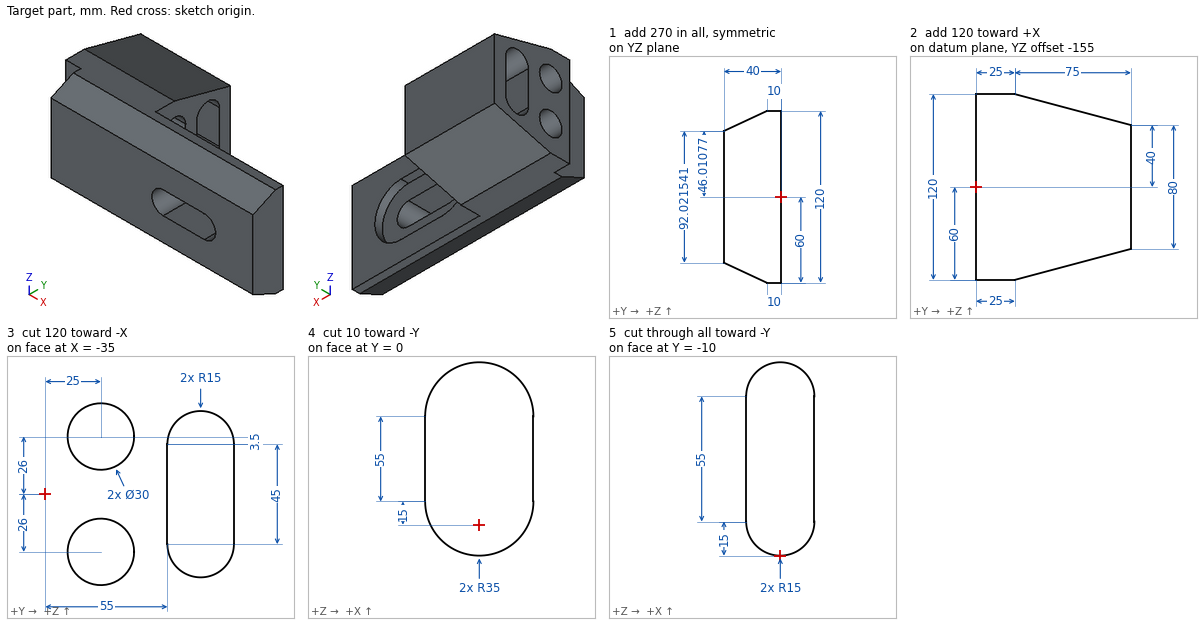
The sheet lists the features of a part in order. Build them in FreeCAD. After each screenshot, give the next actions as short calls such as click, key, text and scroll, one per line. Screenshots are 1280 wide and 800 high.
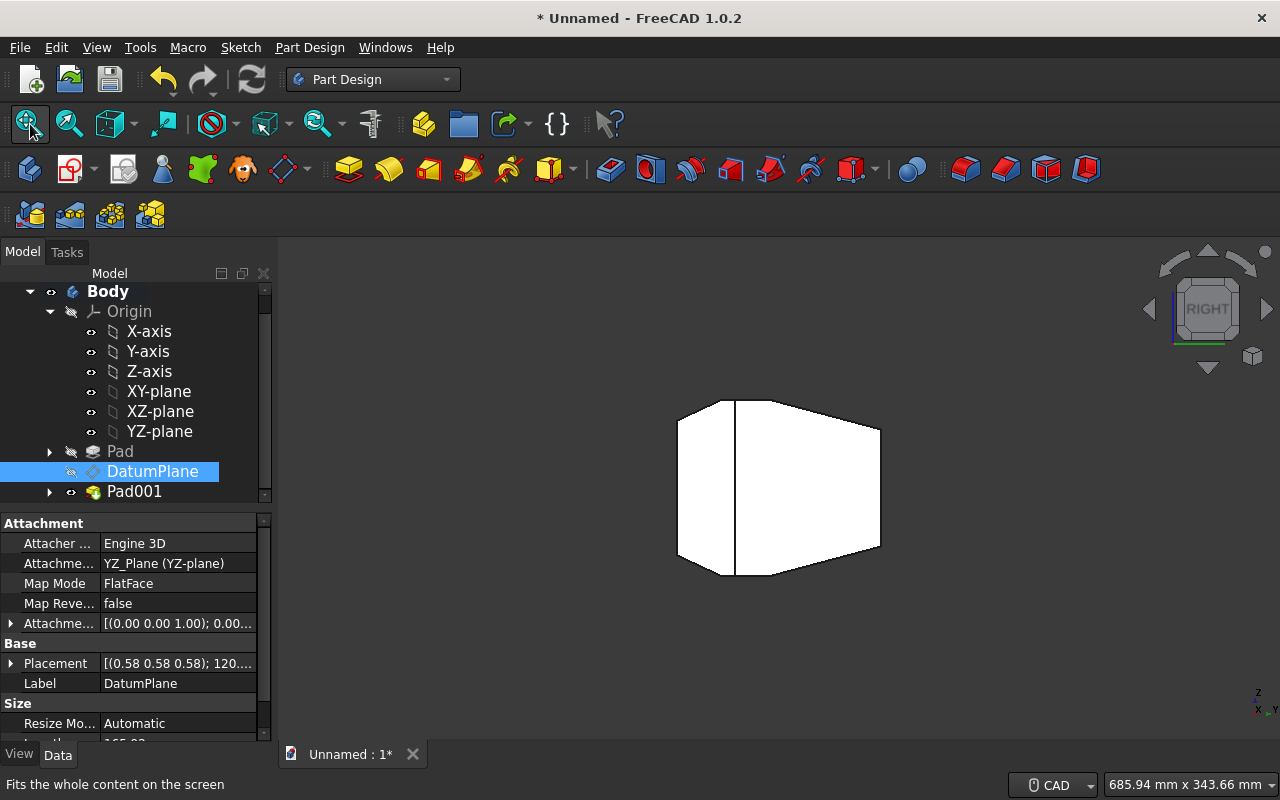
click(808, 487)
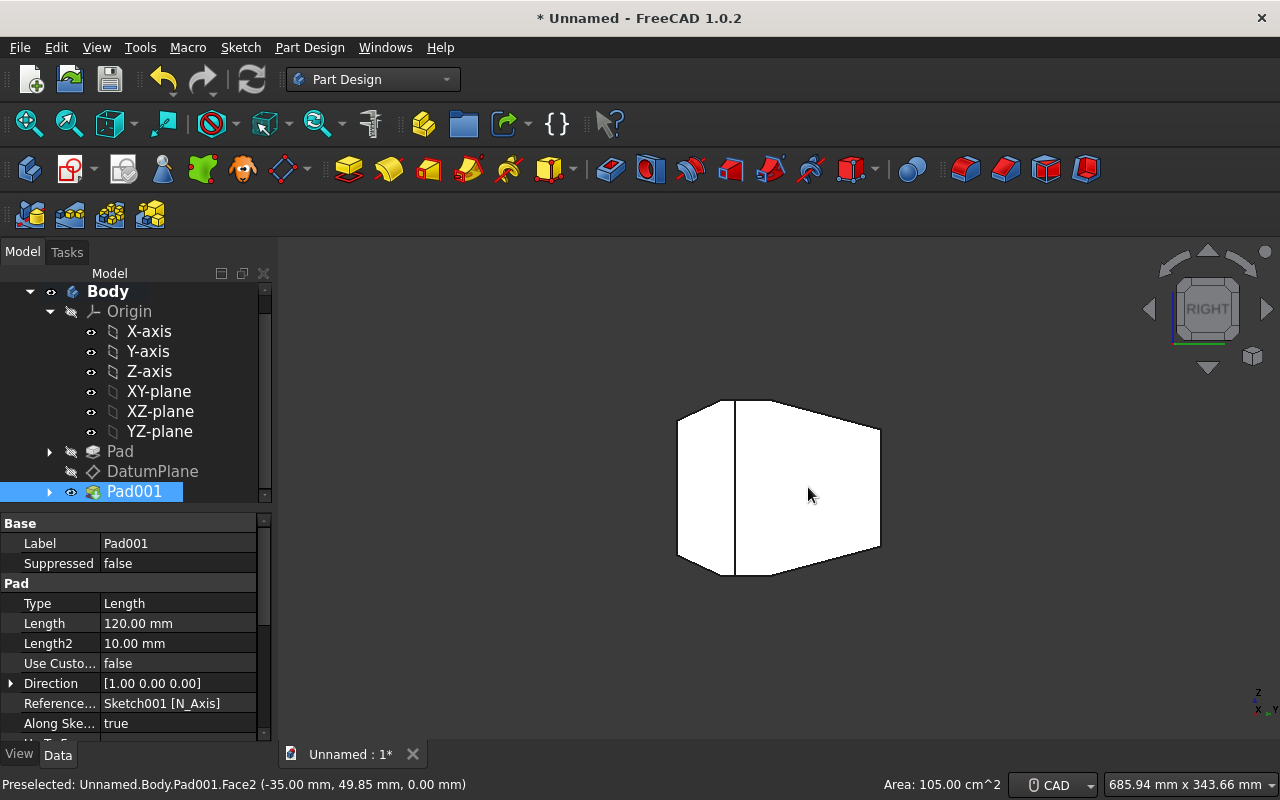
click(70, 170)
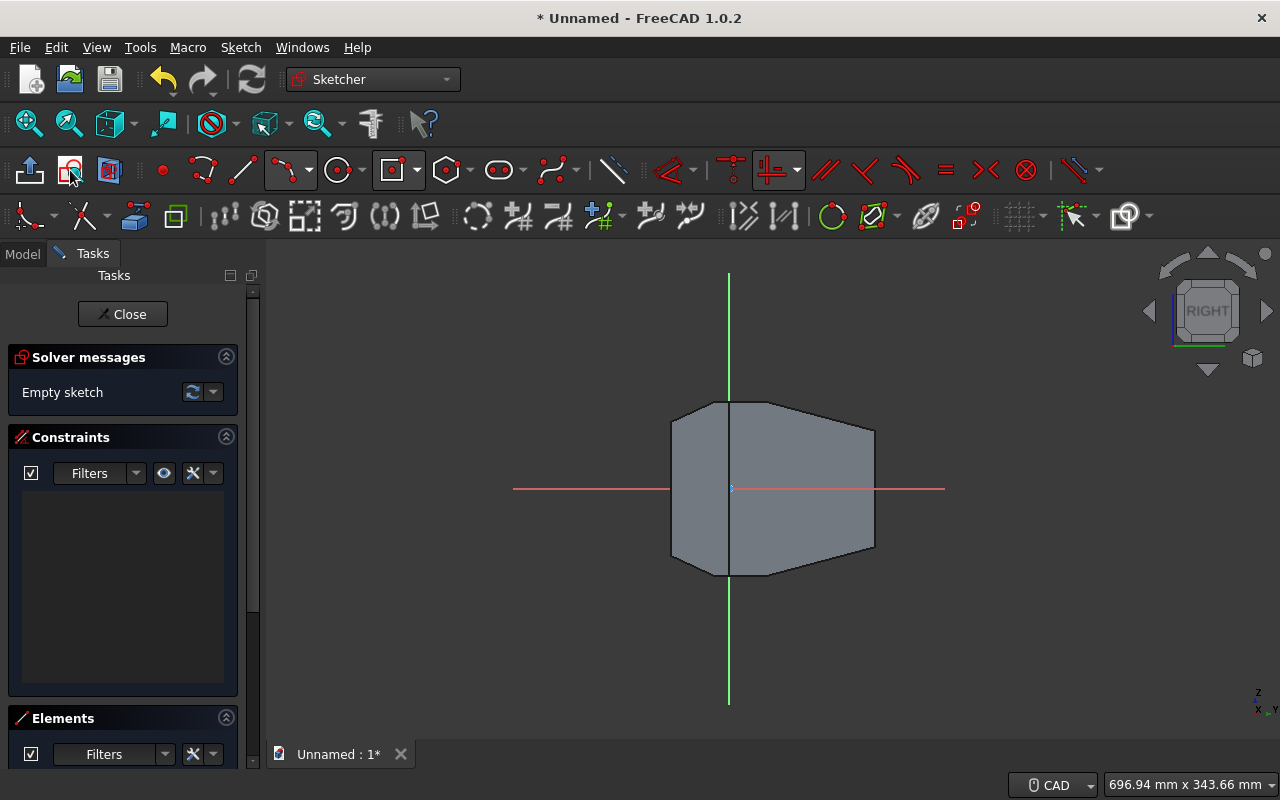
scroll(842, 489, up, 5)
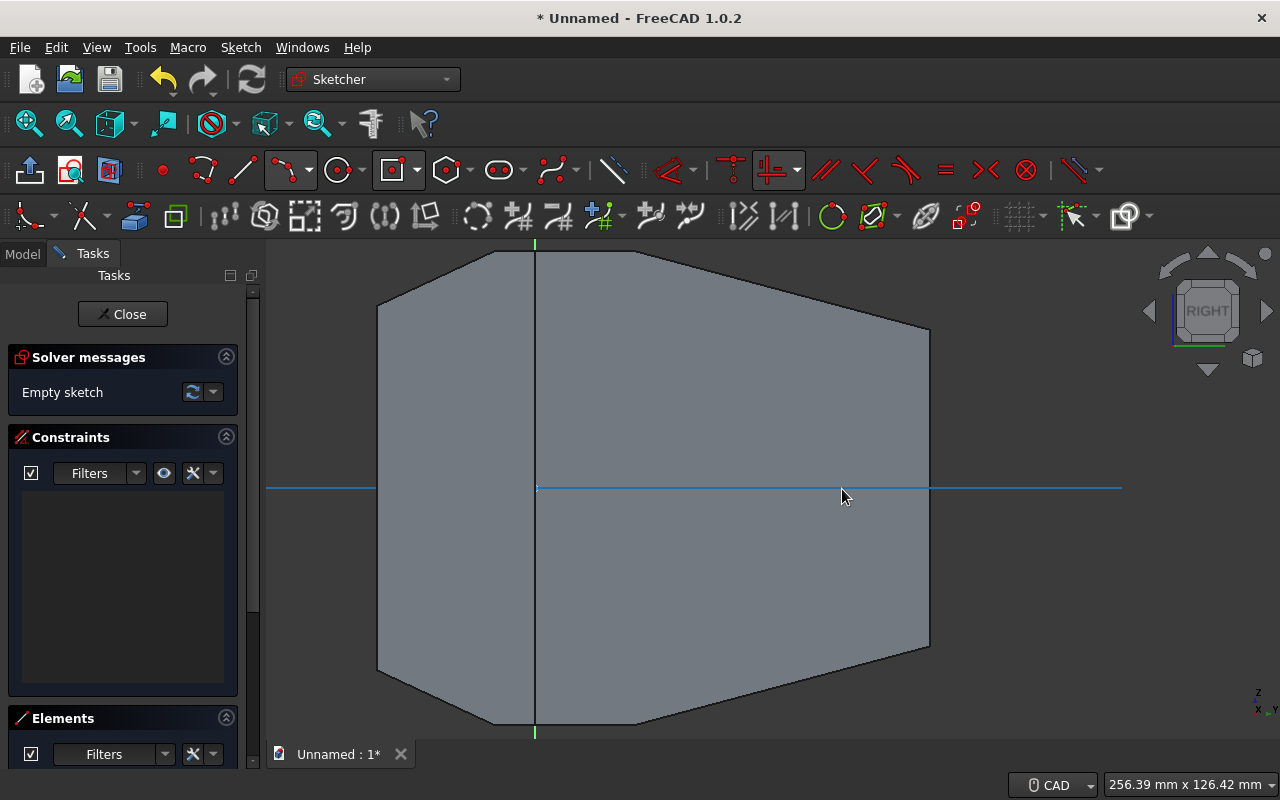
click(500, 170)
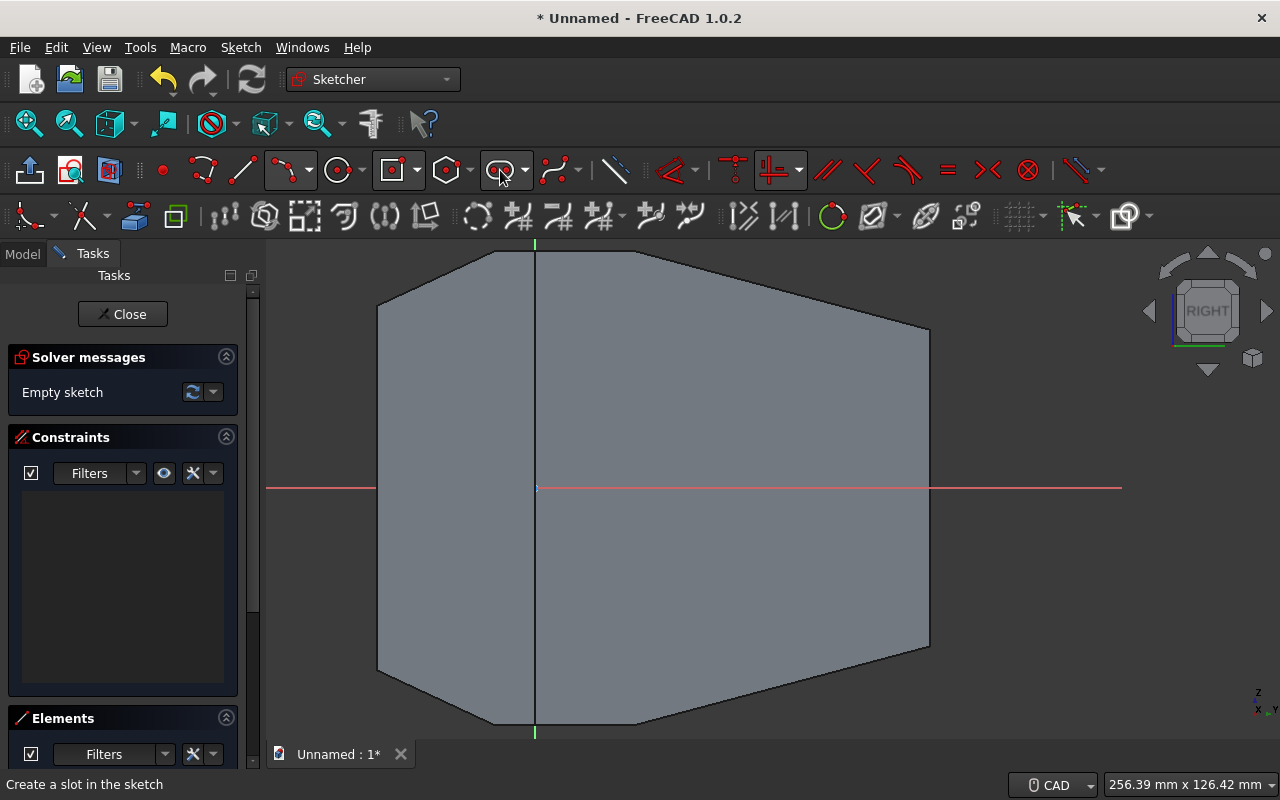
click(812, 577)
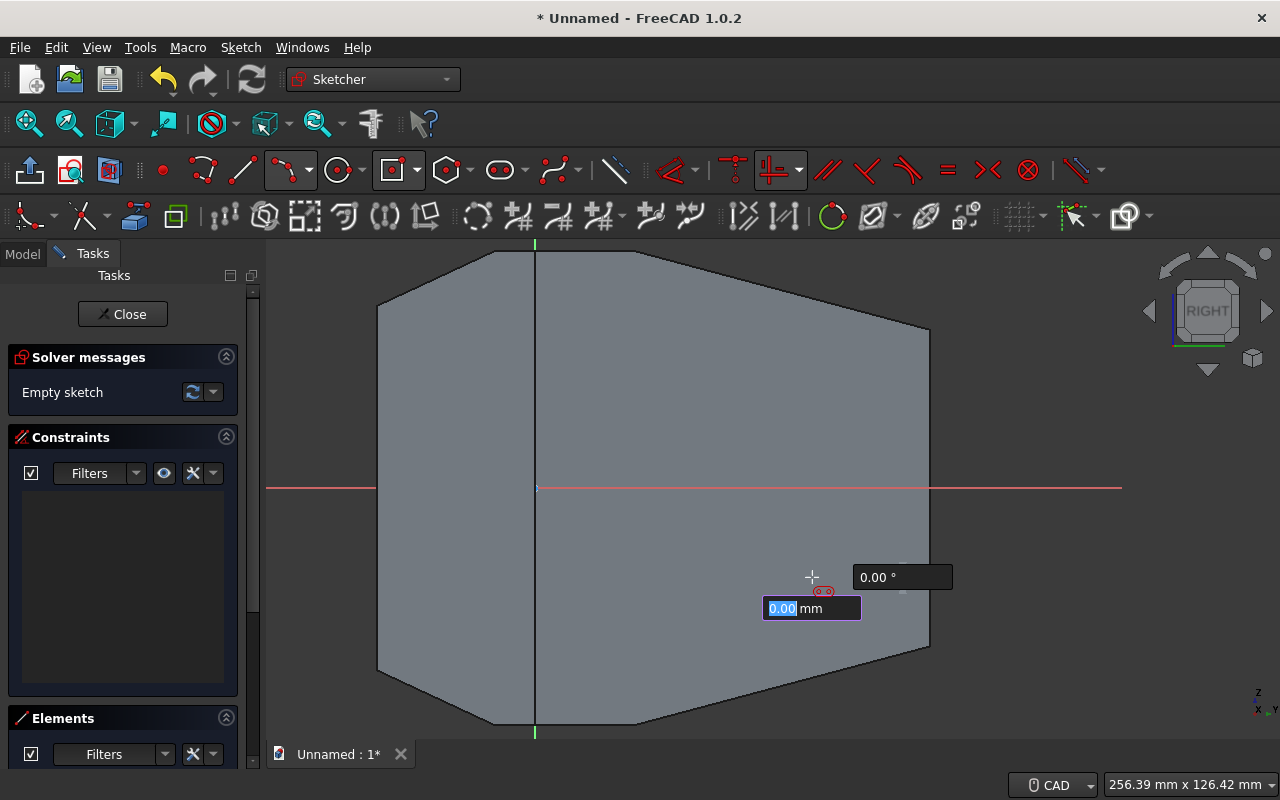
click(812, 399)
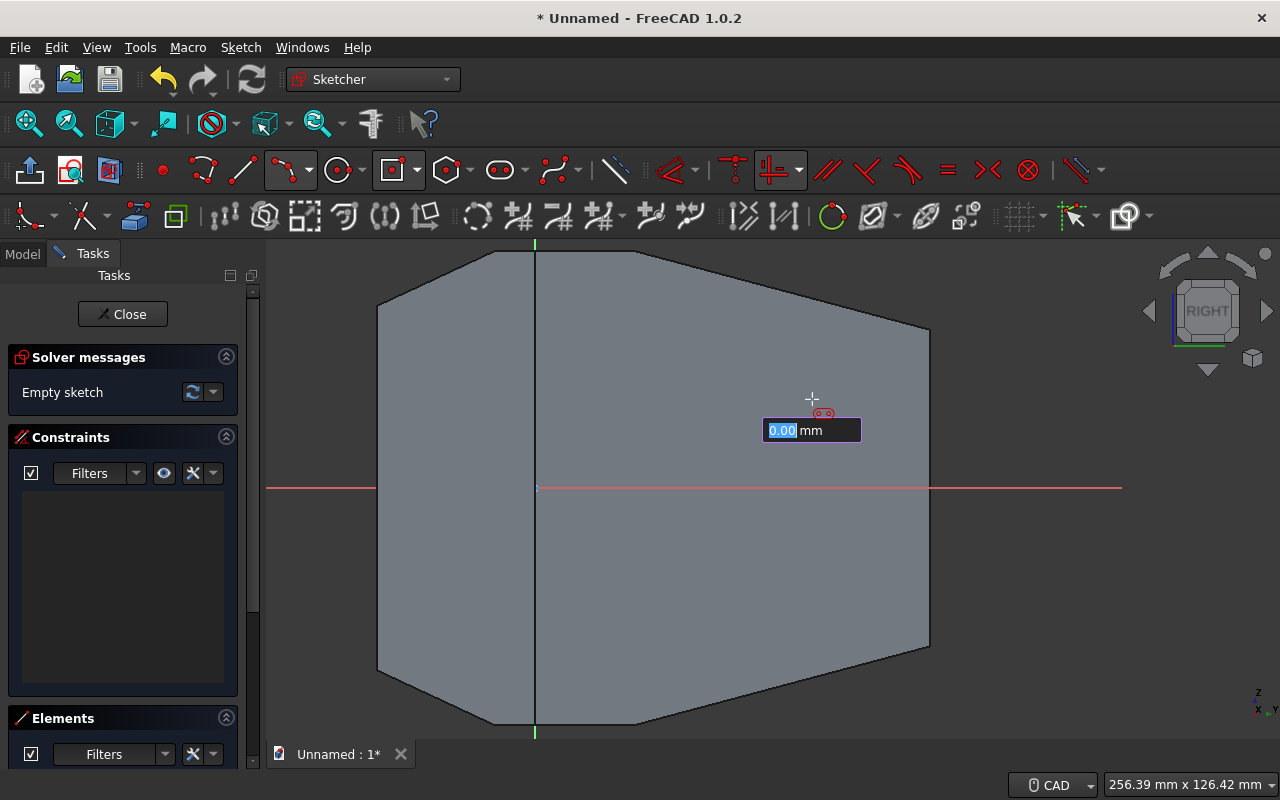
click(871, 515)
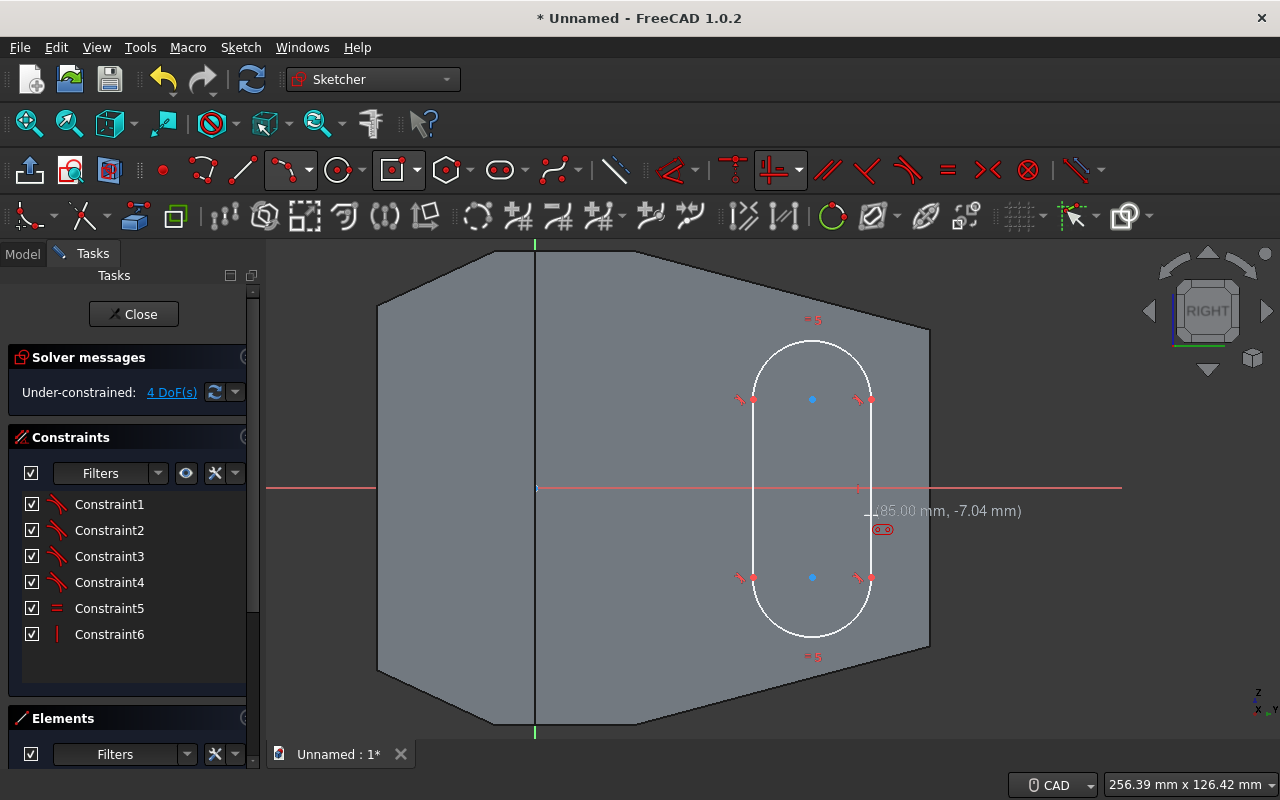
click(338, 170)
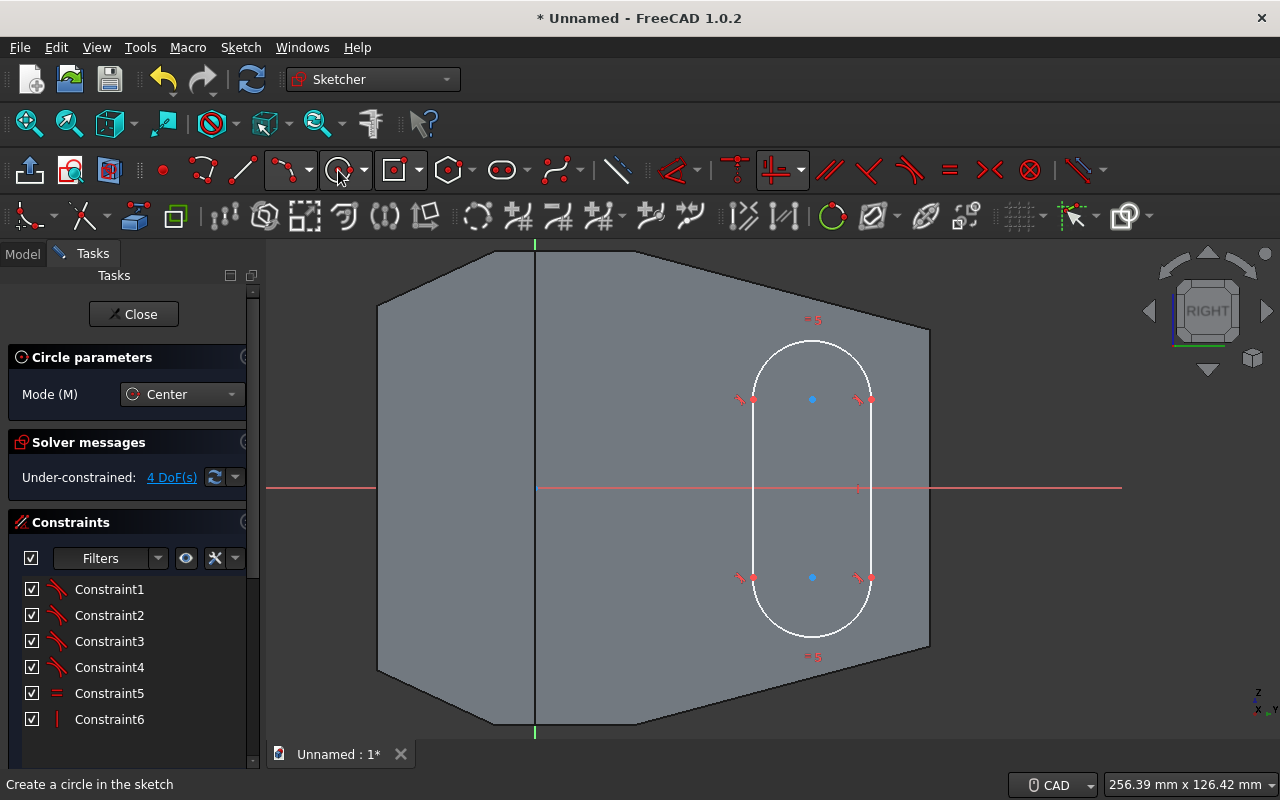
click(634, 385)
click(676, 343)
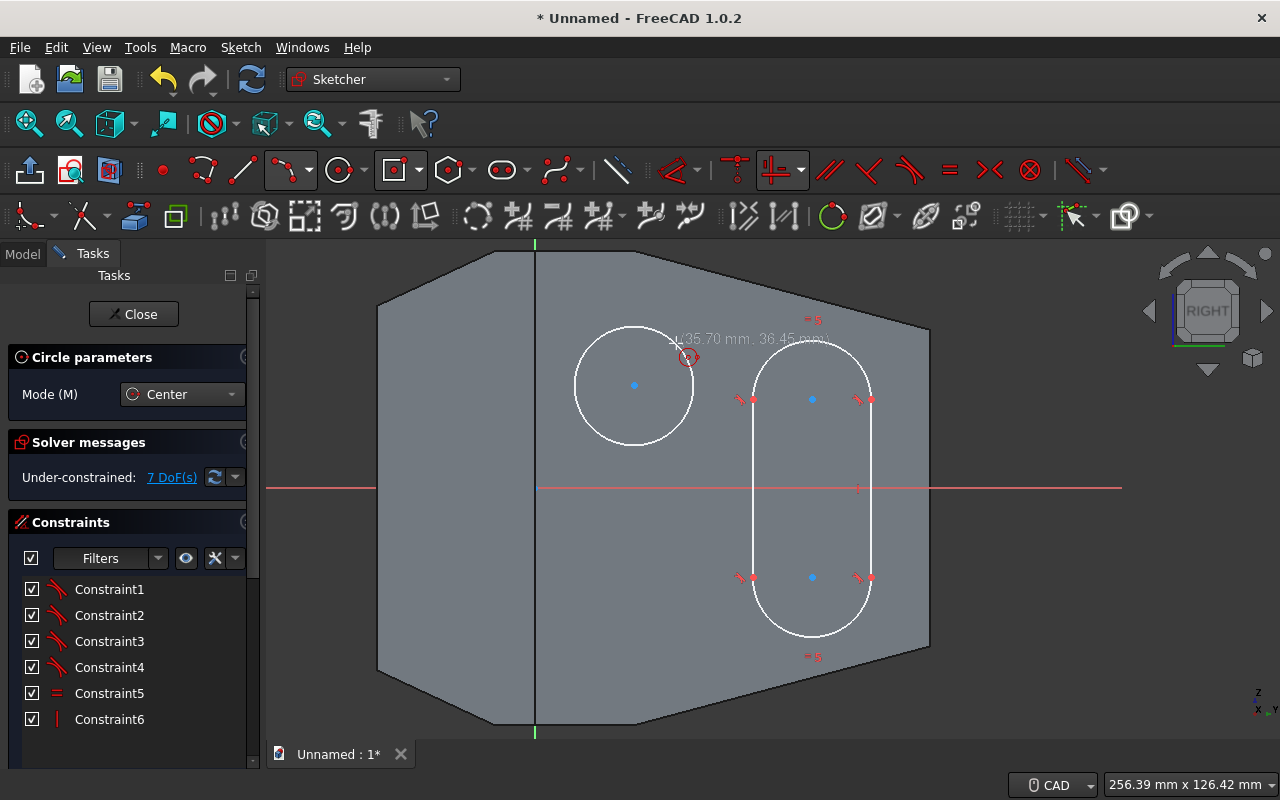
click(634, 591)
click(676, 549)
key(Escape)